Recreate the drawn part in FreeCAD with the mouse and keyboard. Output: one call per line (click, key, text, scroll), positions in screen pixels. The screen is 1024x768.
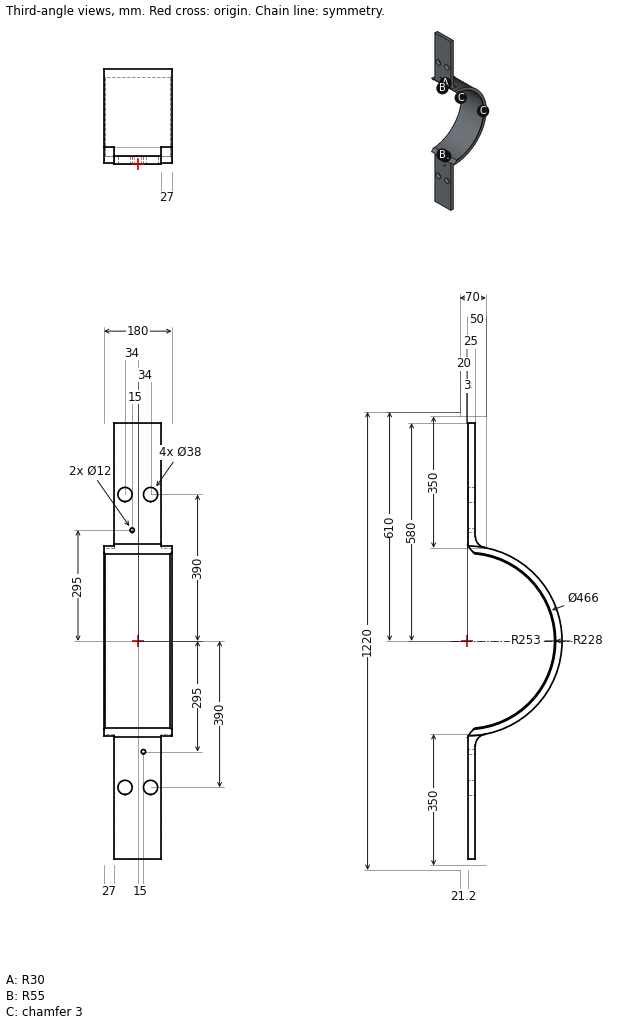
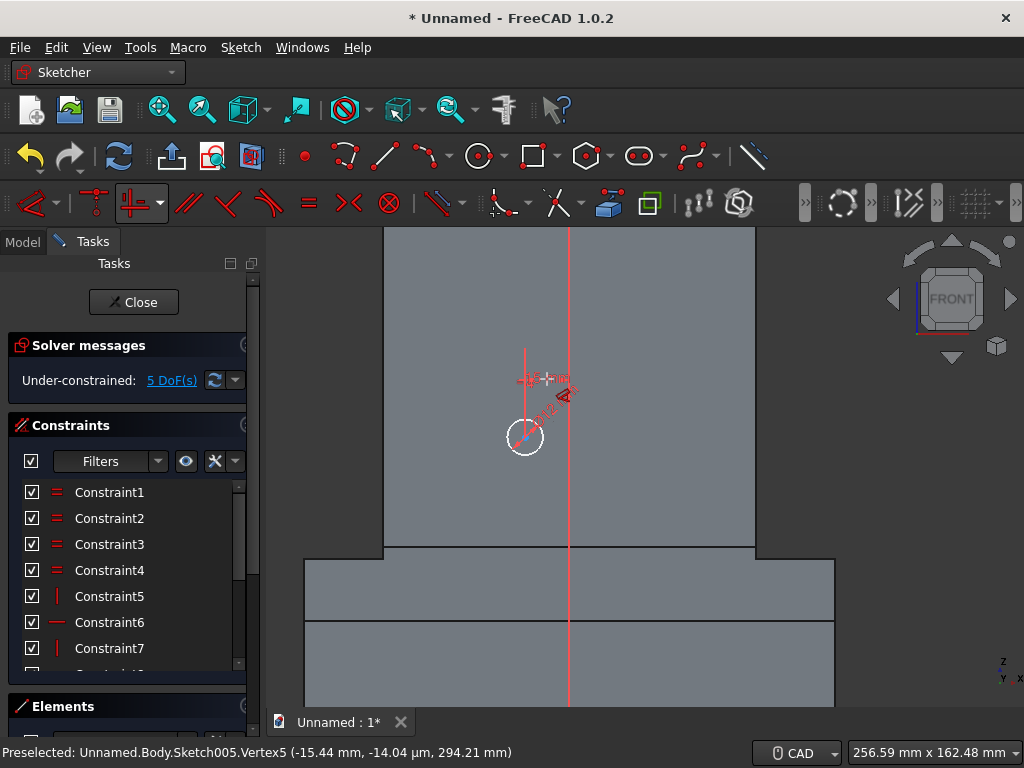
scroll(578, 336, down, 10)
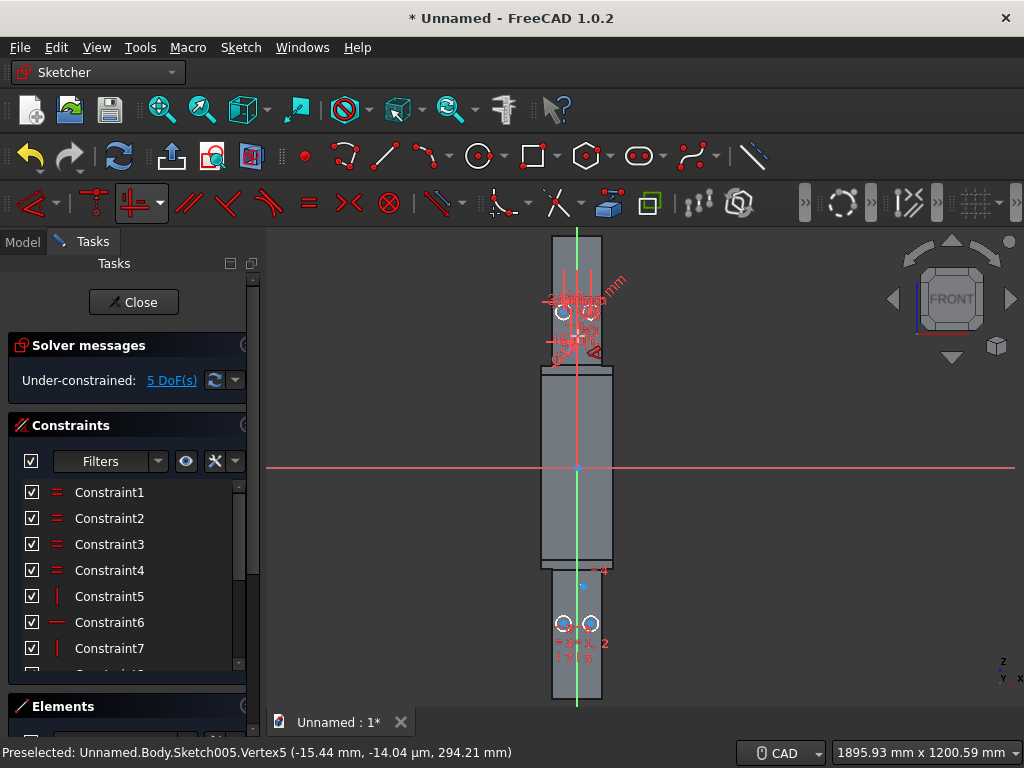
scroll(583, 586, up, 10)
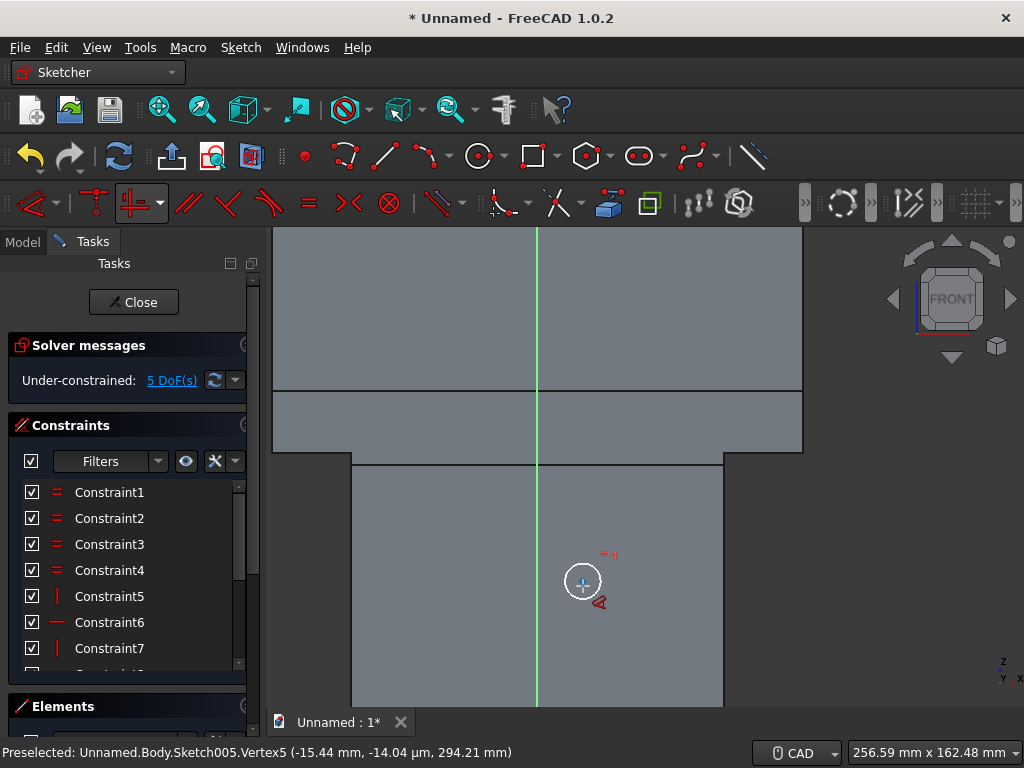
click(583, 581)
click(560, 615)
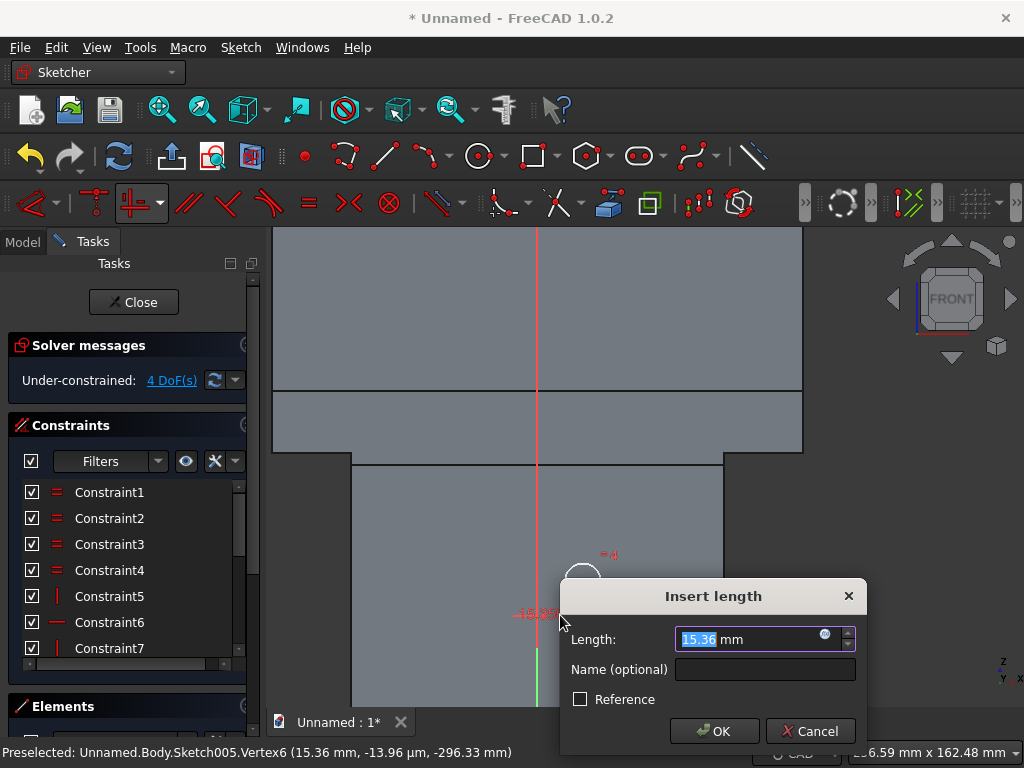
text(15)
key(Return)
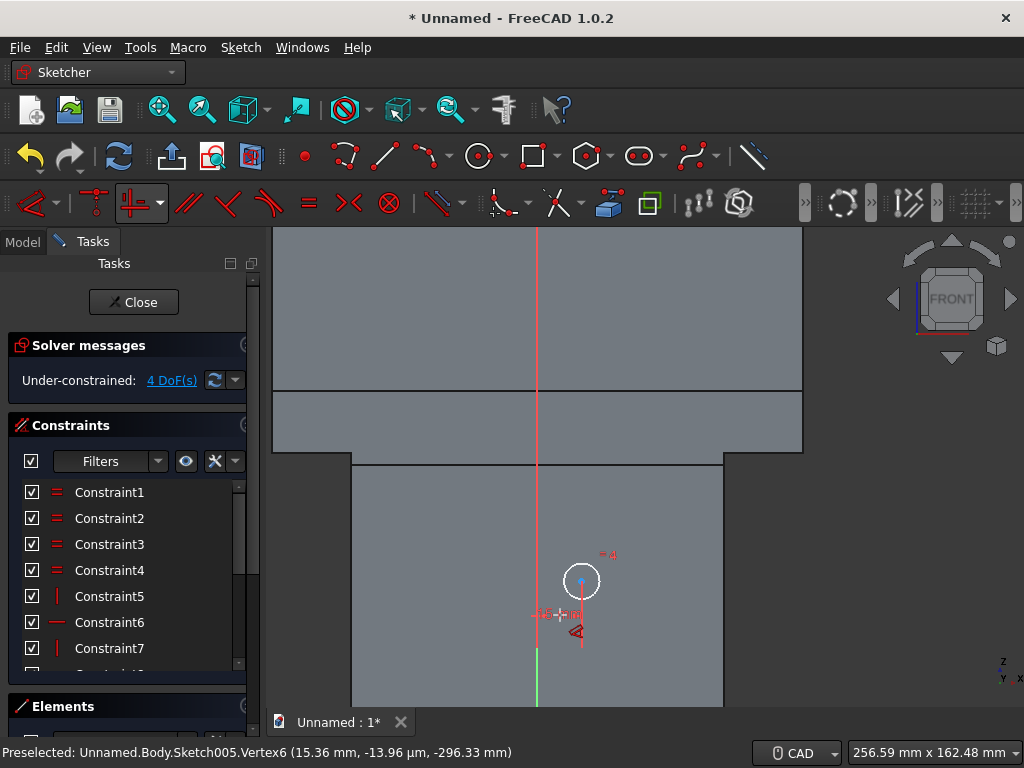
scroll(583, 586, down, 10)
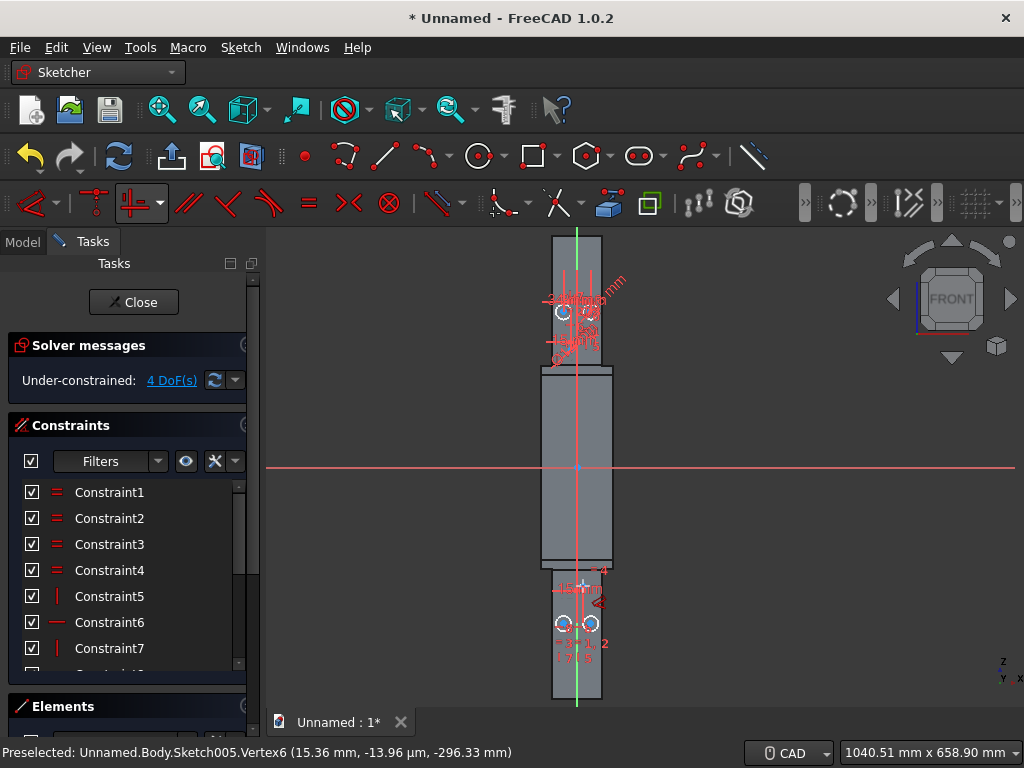
click(591, 312)
click(625, 390)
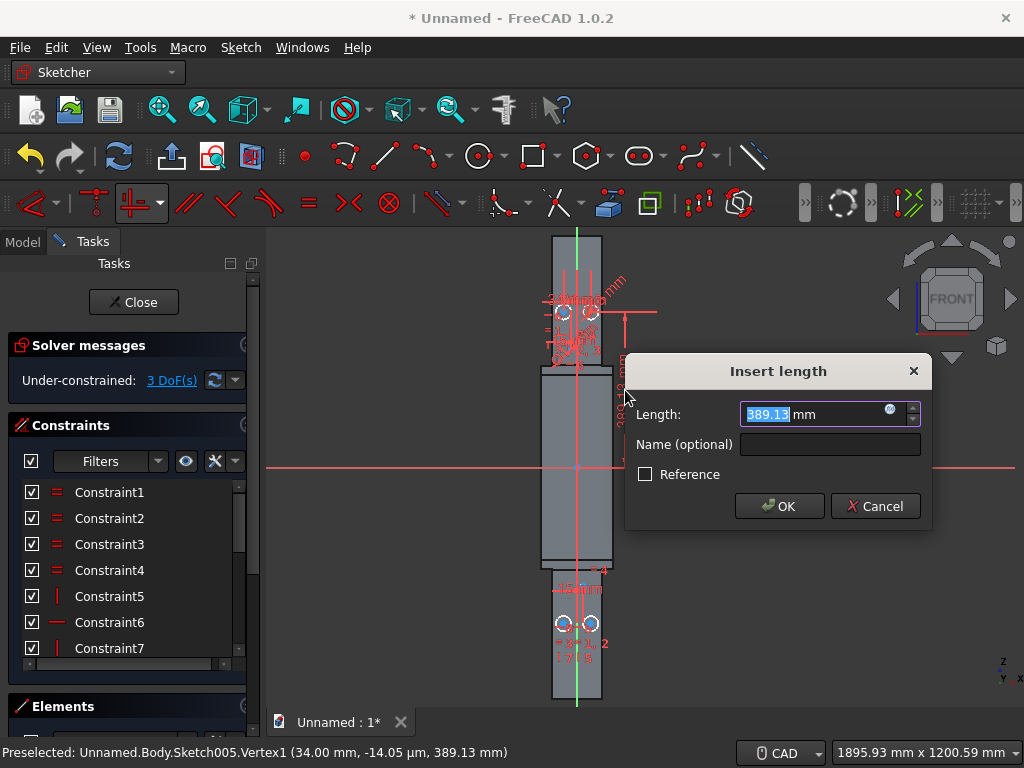
text(390)
key(Return)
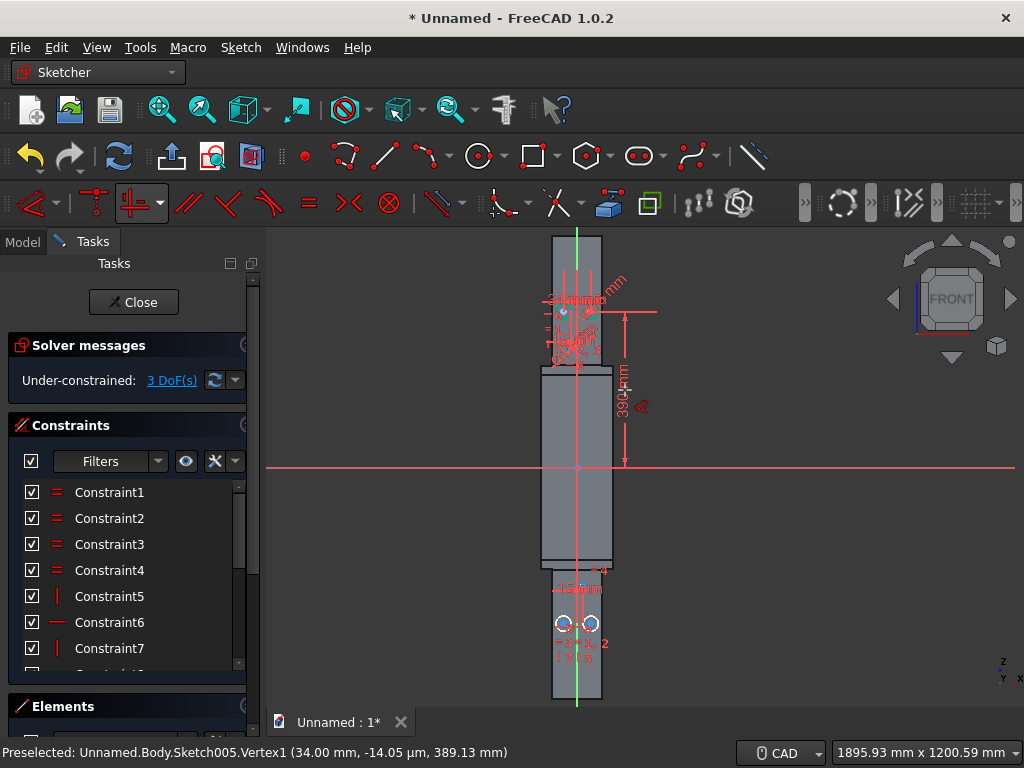
click(591, 624)
click(625, 546)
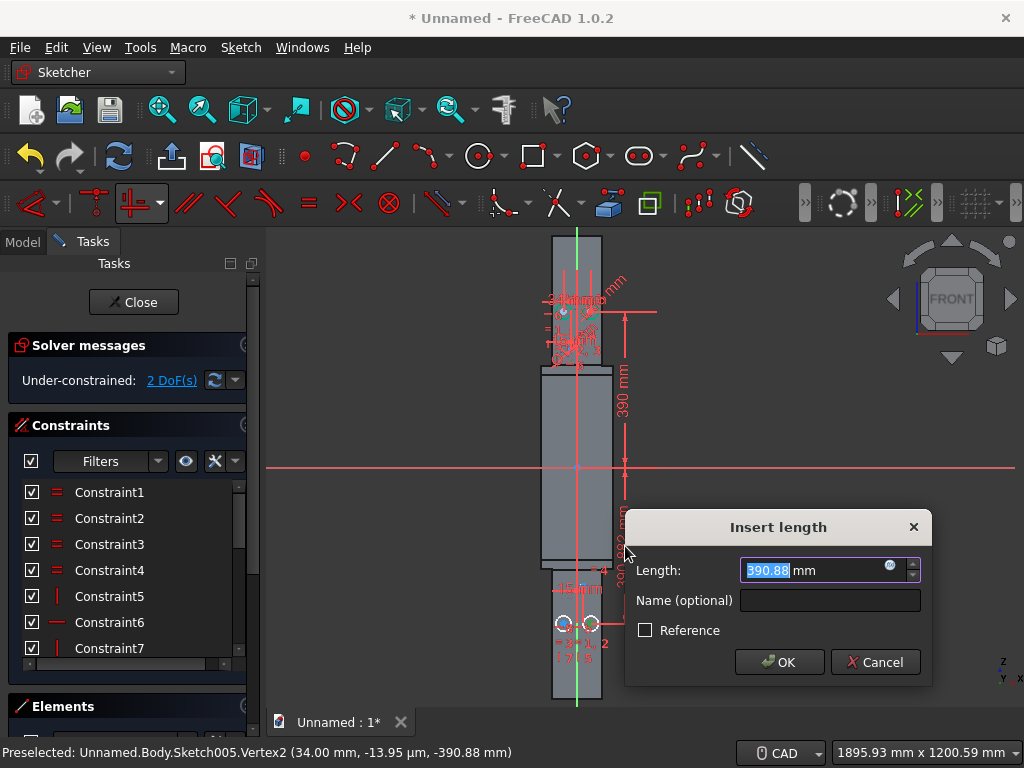
text(390)
key(Return)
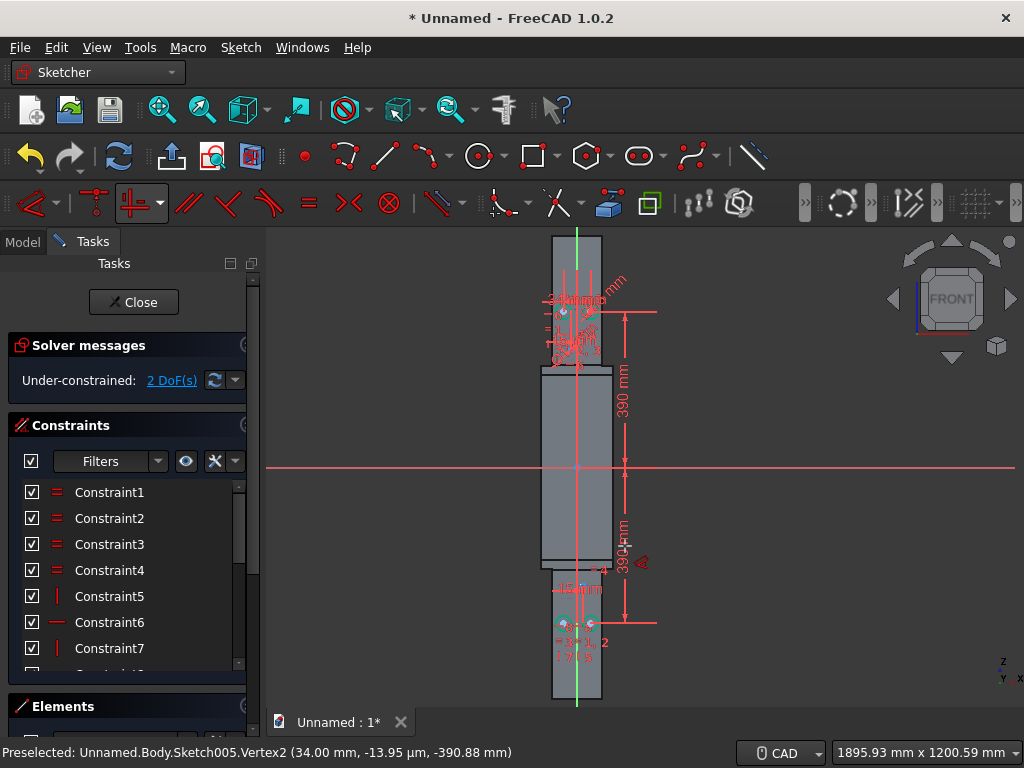
click(571, 350)
click(537, 409)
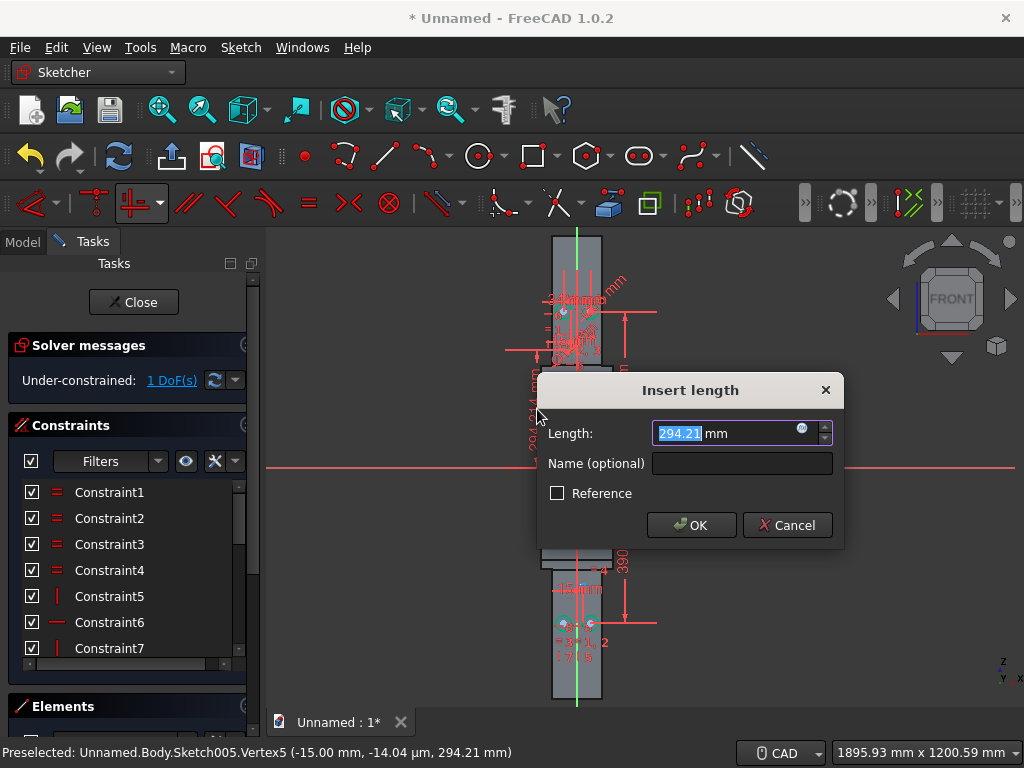
text(295)
key(Return)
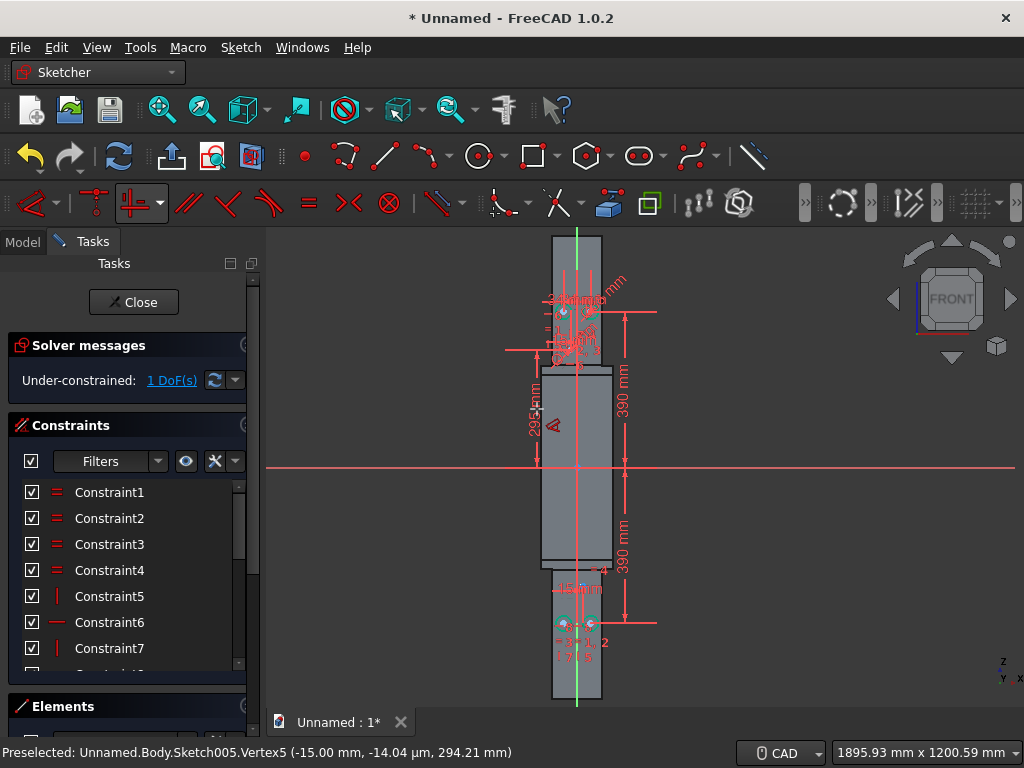
click(583, 586)
click(617, 500)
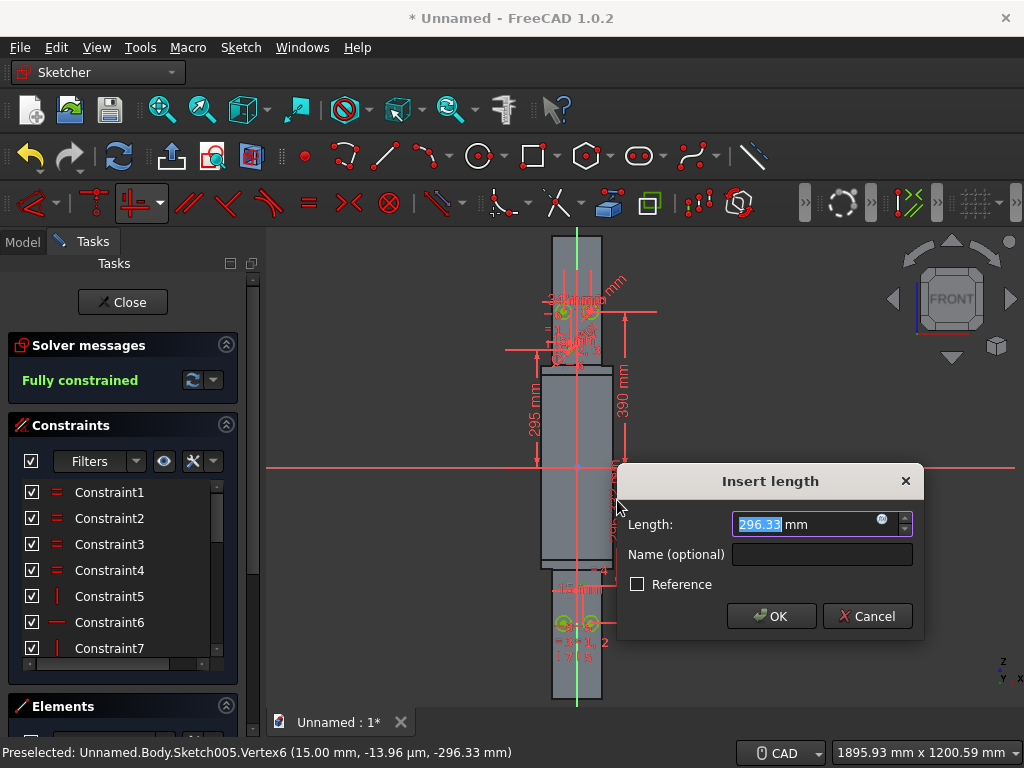
text(295)
key(Return)
key(Escape)